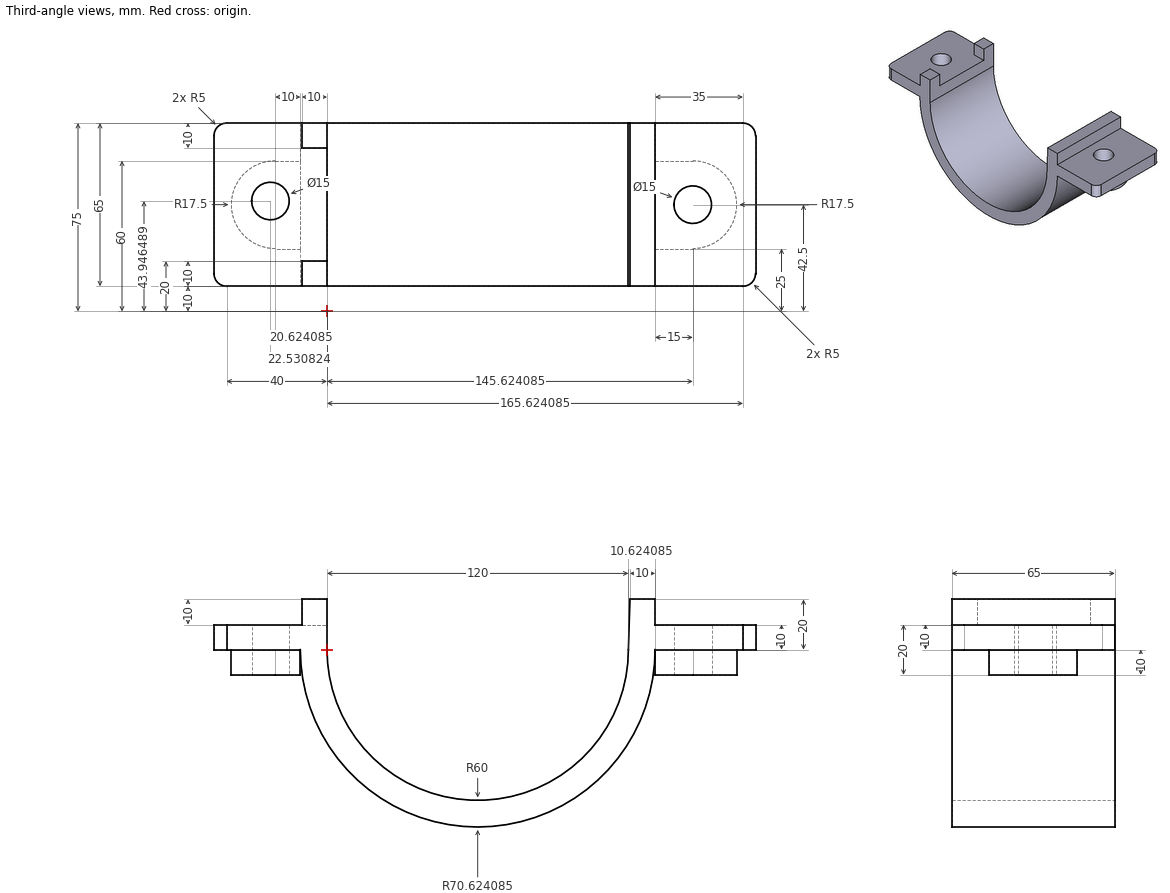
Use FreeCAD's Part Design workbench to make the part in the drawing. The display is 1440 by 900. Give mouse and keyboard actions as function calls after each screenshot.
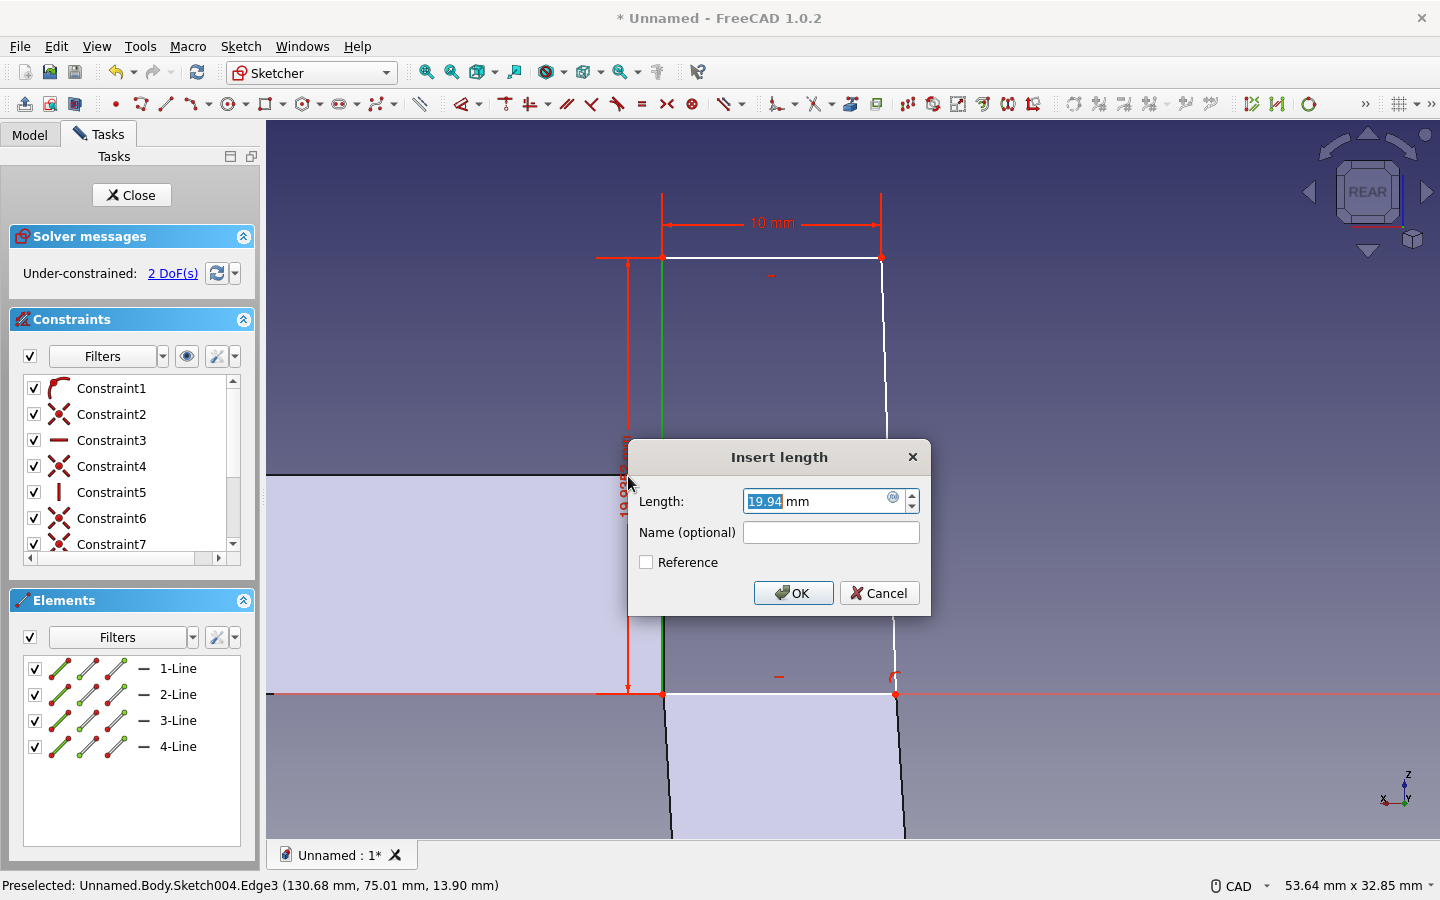
text(20)
key(Return)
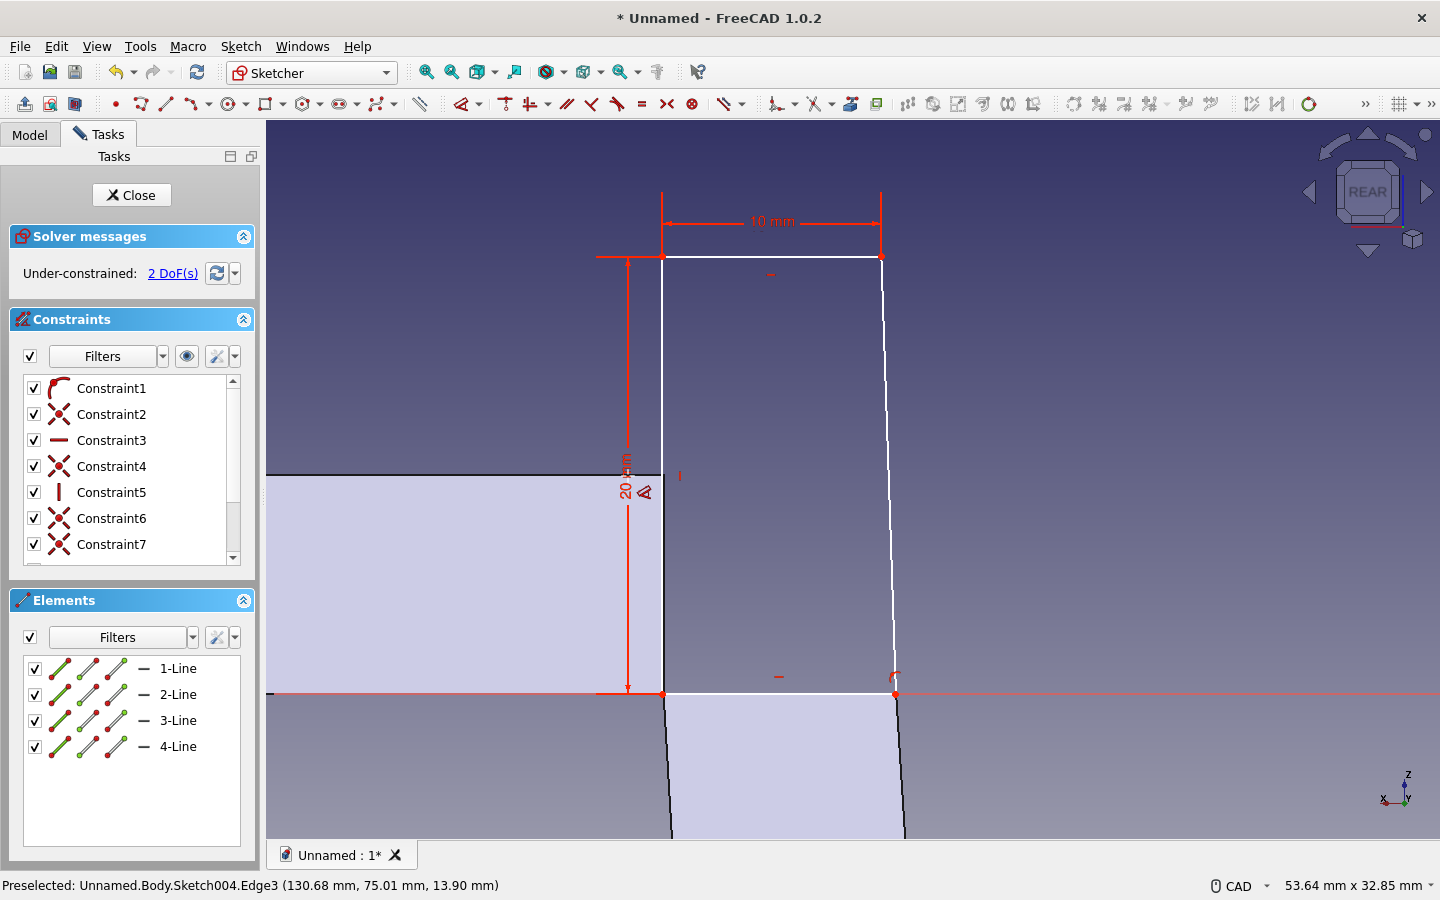
click(896, 694)
click(1086, 728)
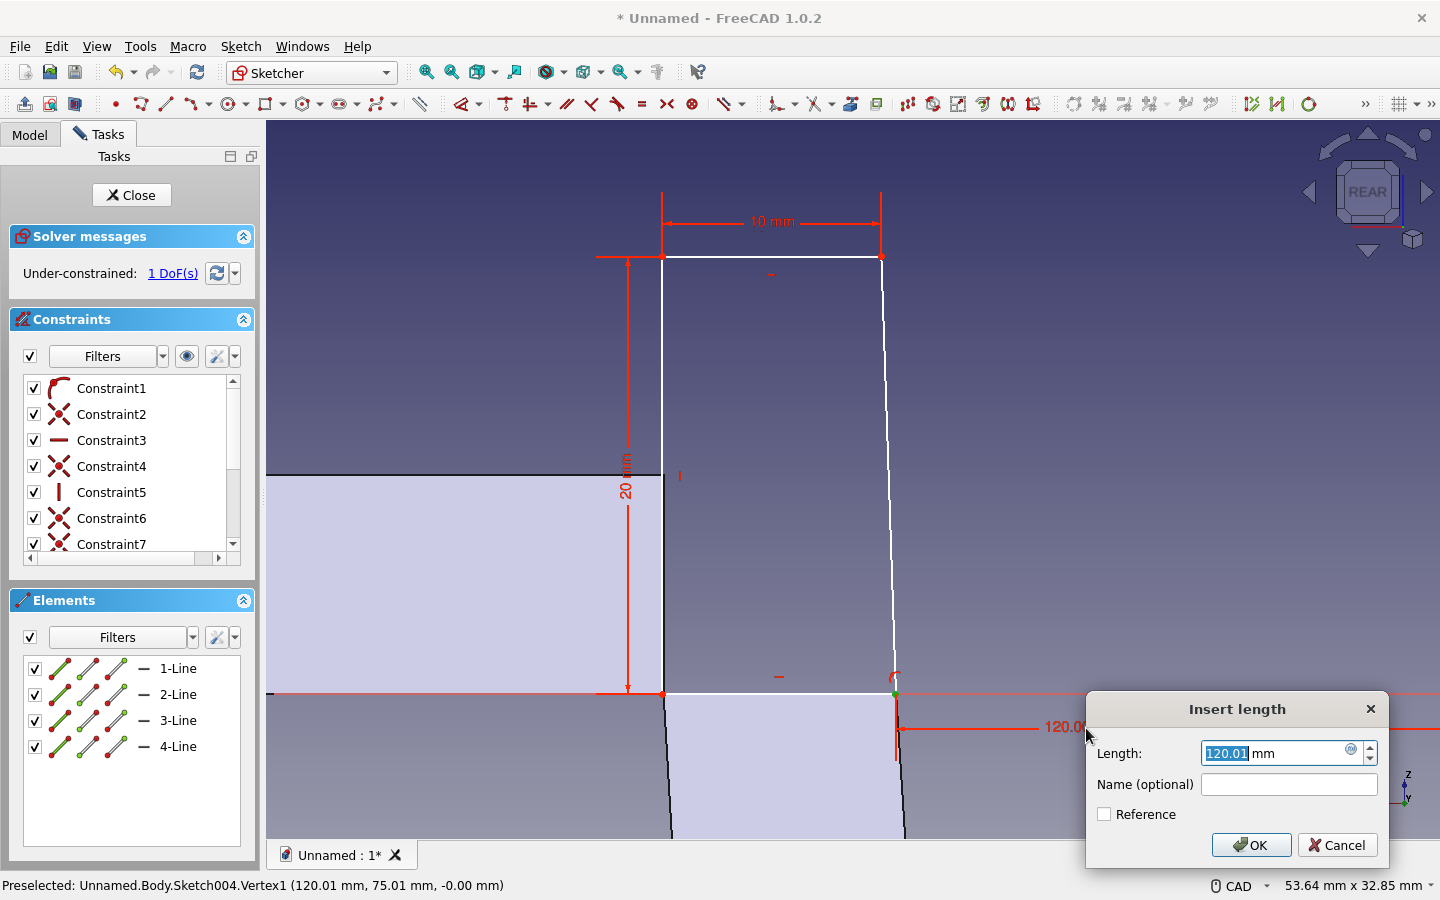
text(120)
key(Return)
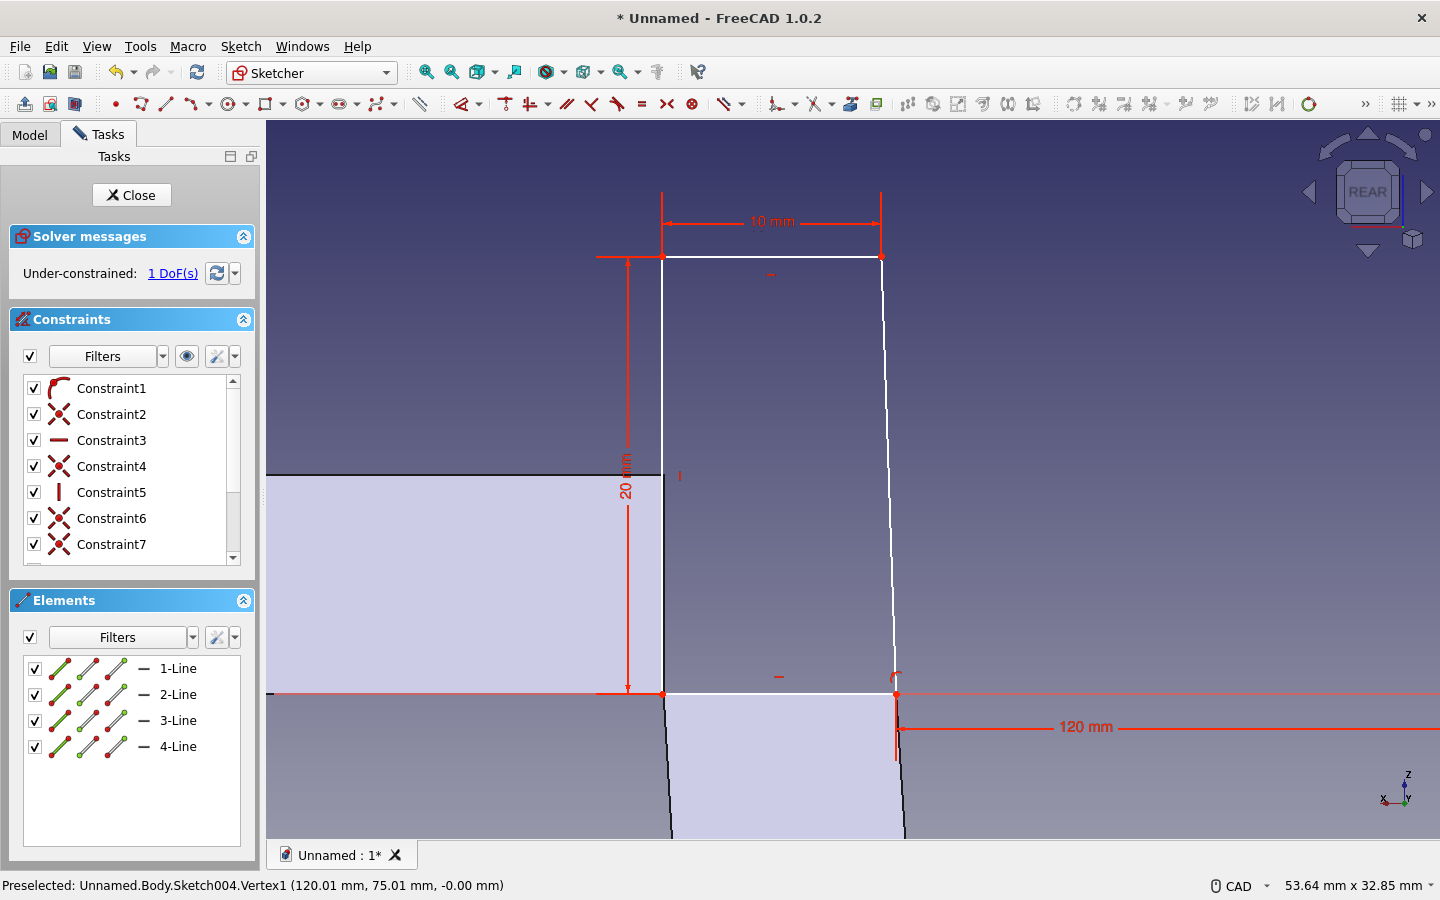
click(733, 694)
click(779, 728)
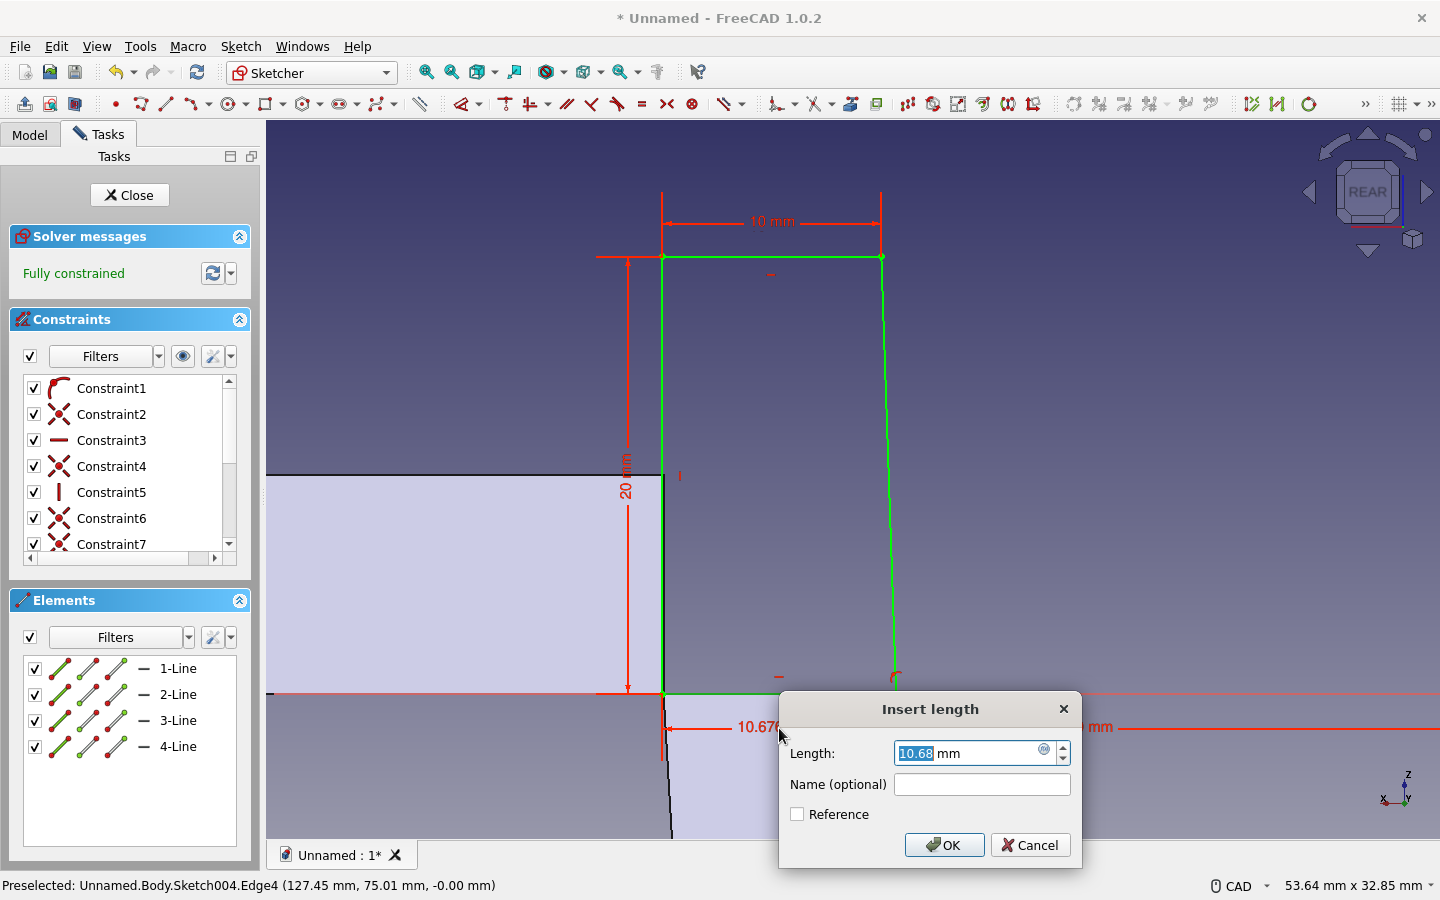
text(10.624085)
key(Return)
key(Escape)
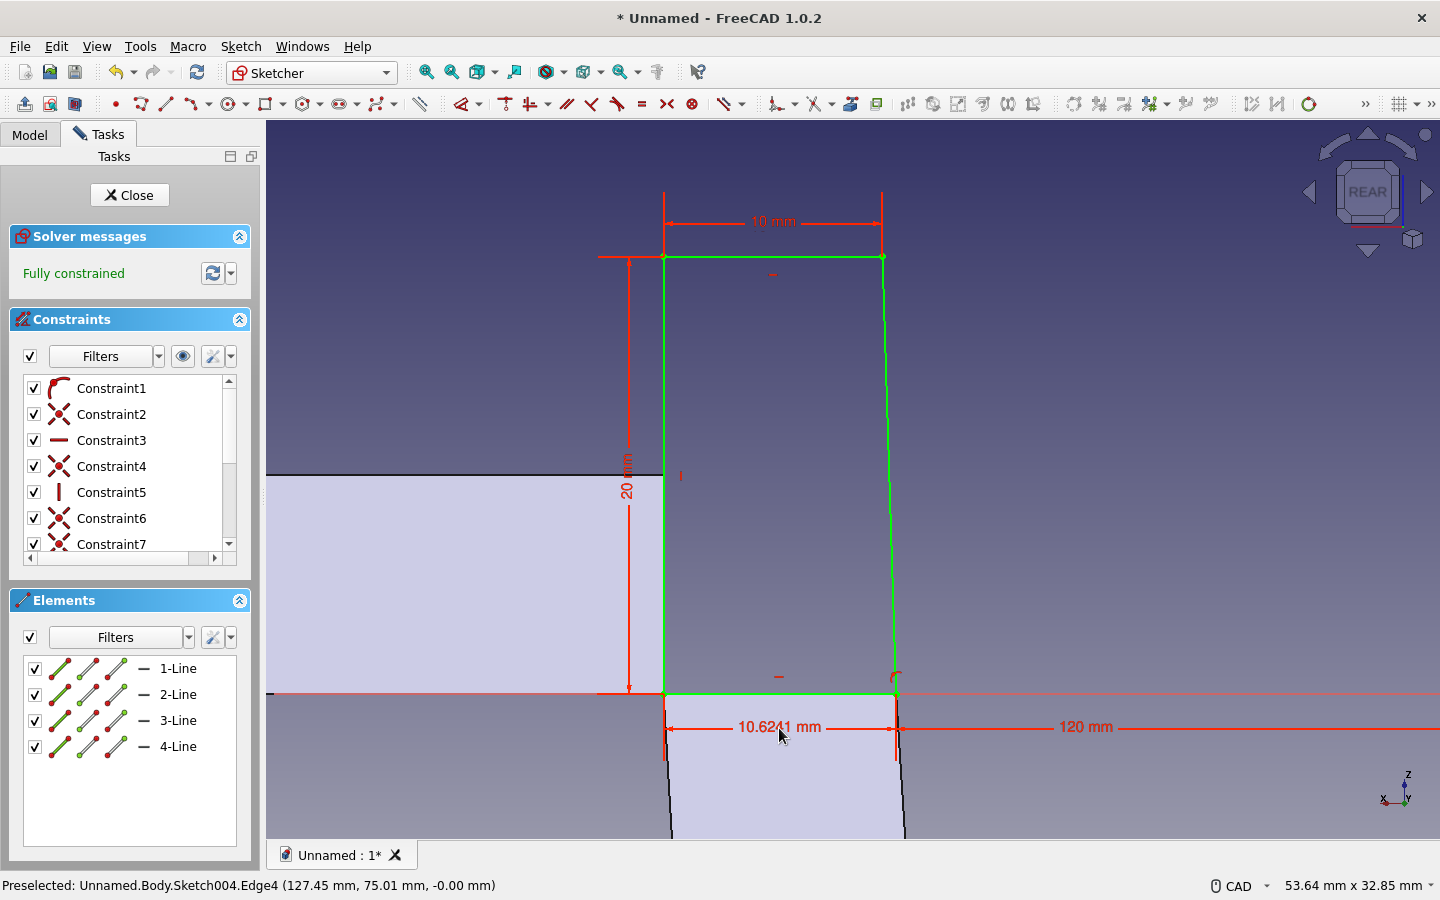
click(130, 195)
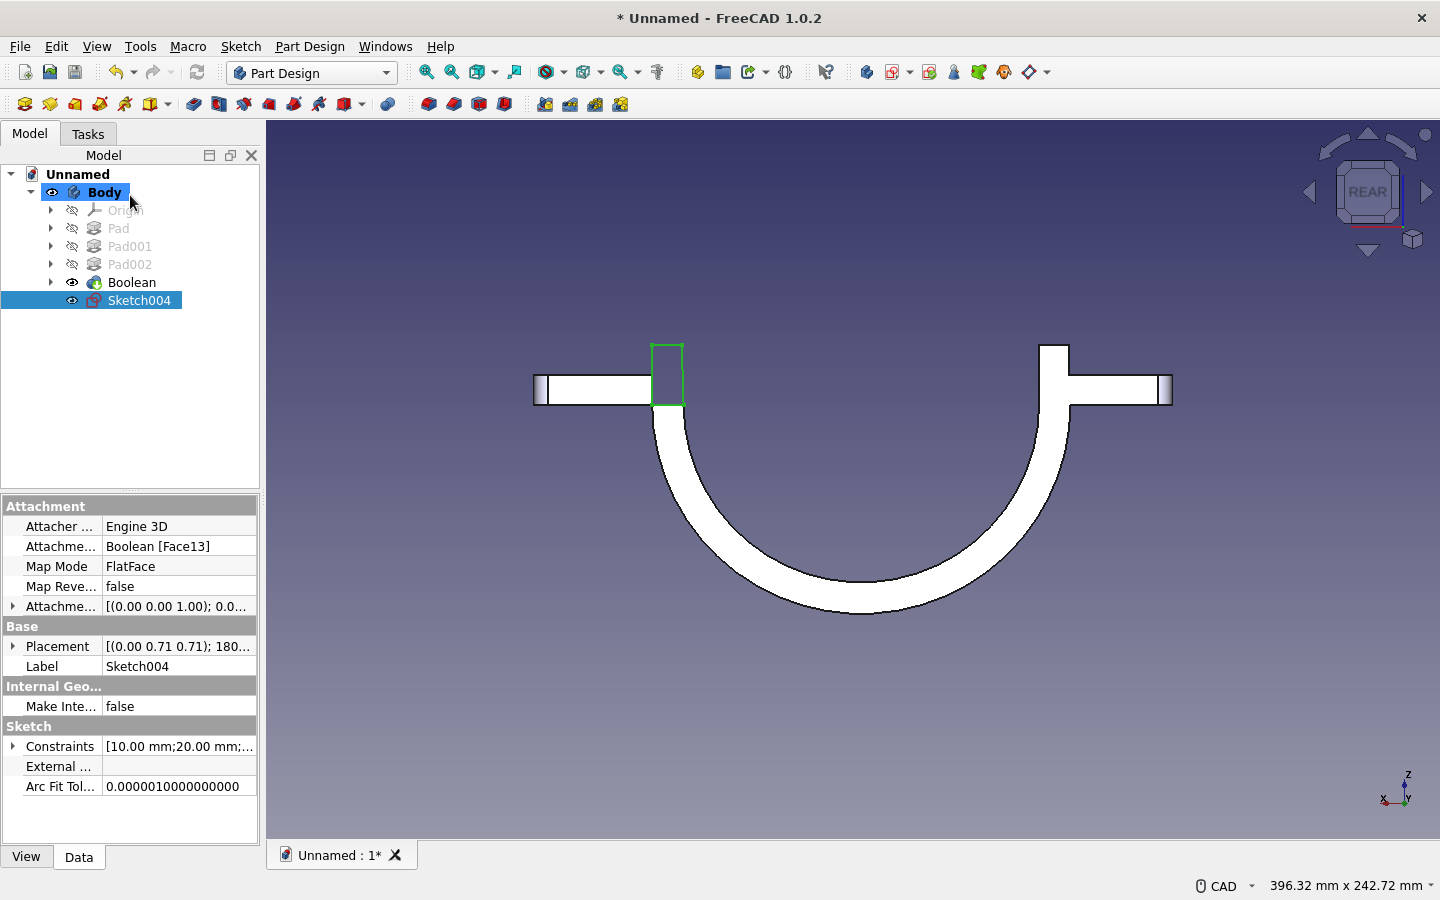
click(25, 104)